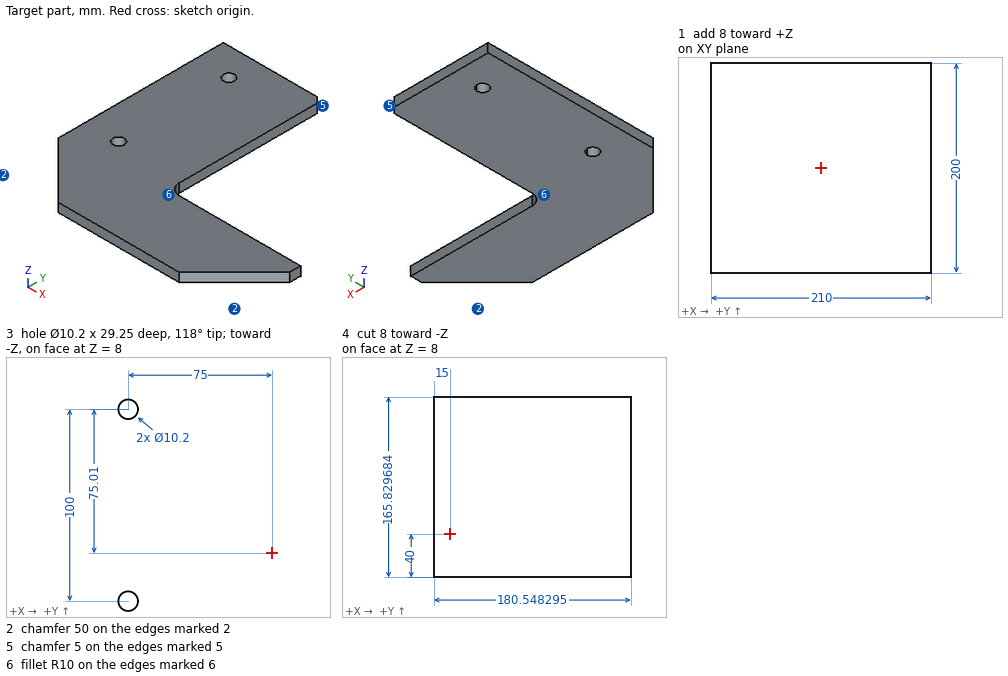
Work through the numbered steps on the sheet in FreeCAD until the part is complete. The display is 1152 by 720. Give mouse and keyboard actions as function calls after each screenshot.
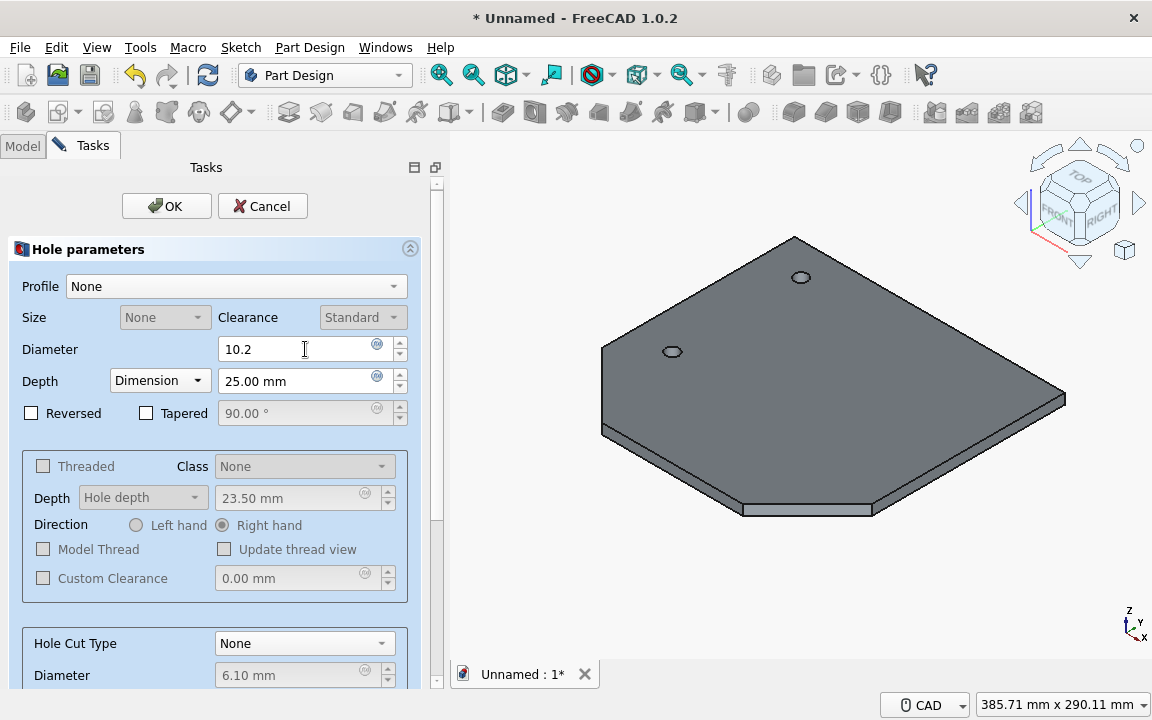
triple_click(305, 381)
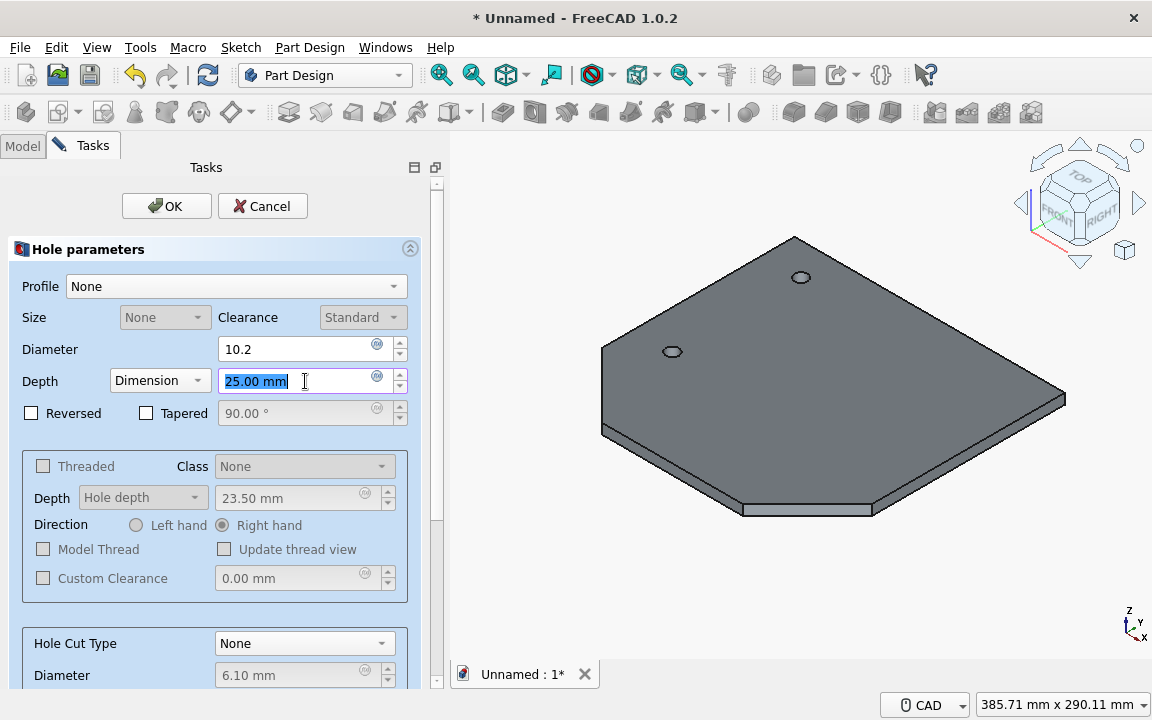
text(29.25)
key(Tab)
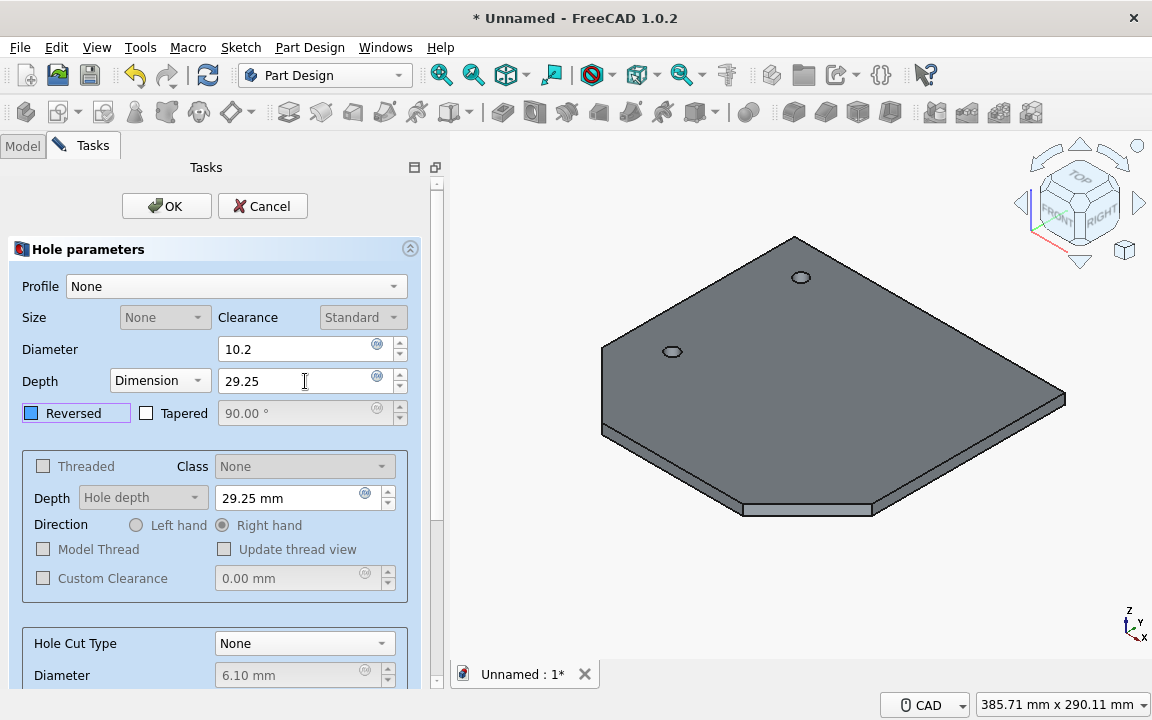
click(167, 206)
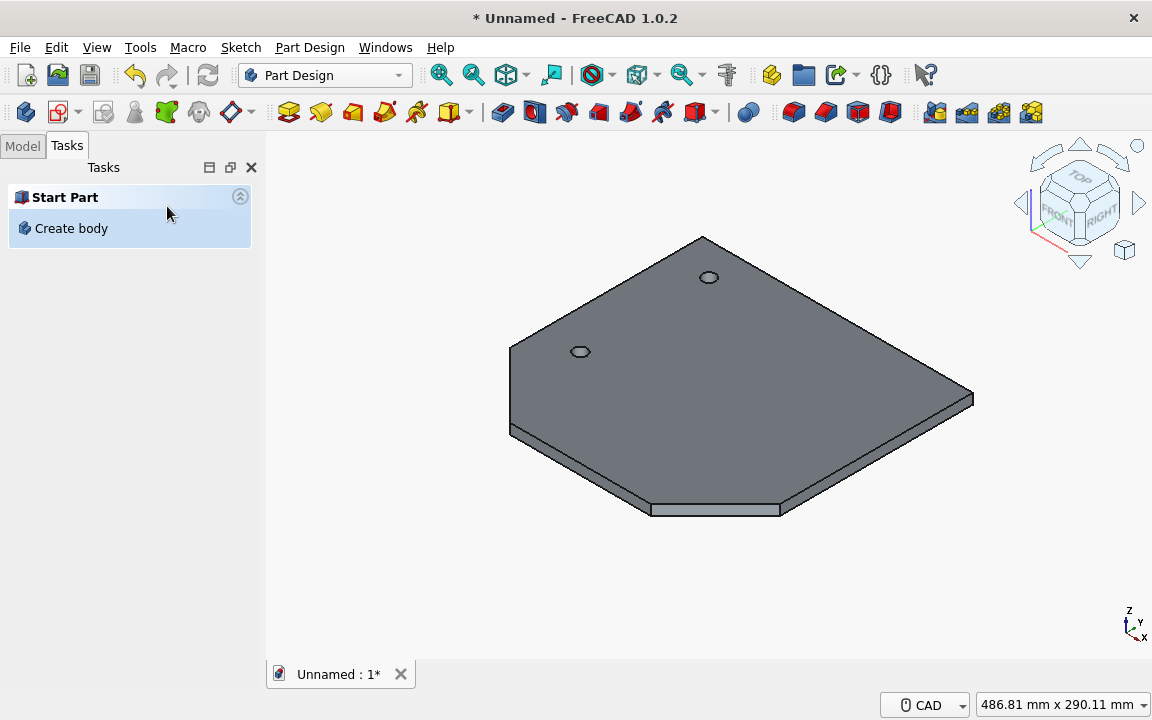
click(748, 410)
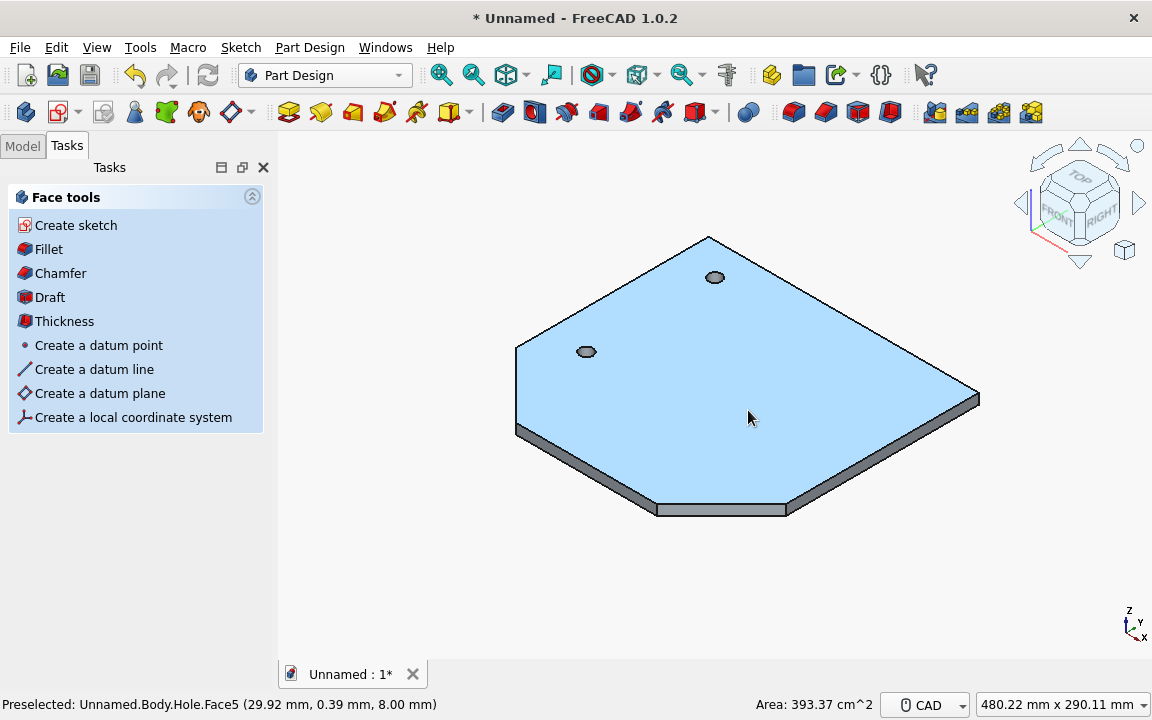
click(58, 112)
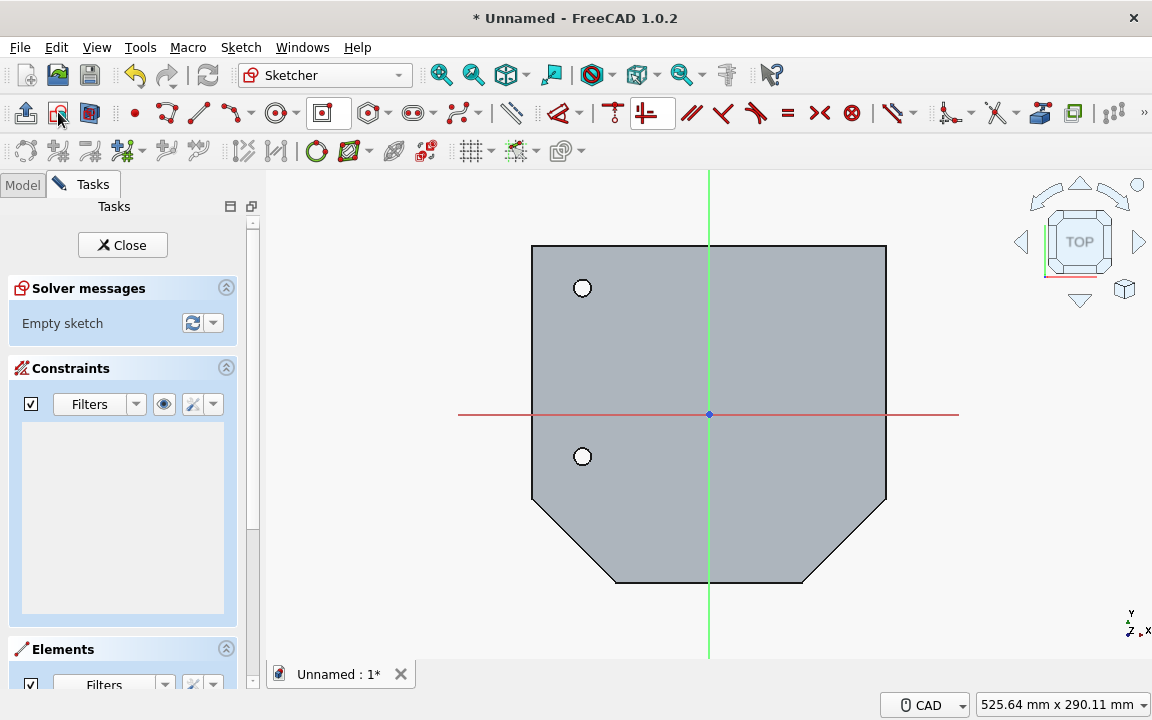
scroll(294, 631, down, 1)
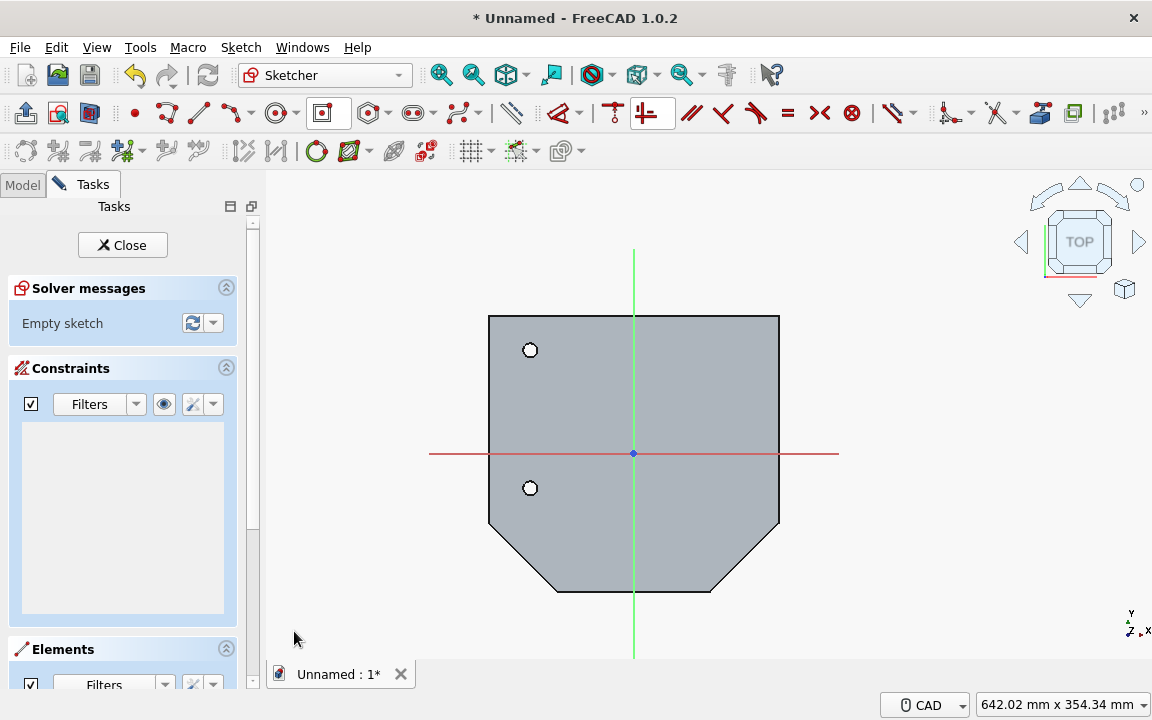
key(g)
key(r)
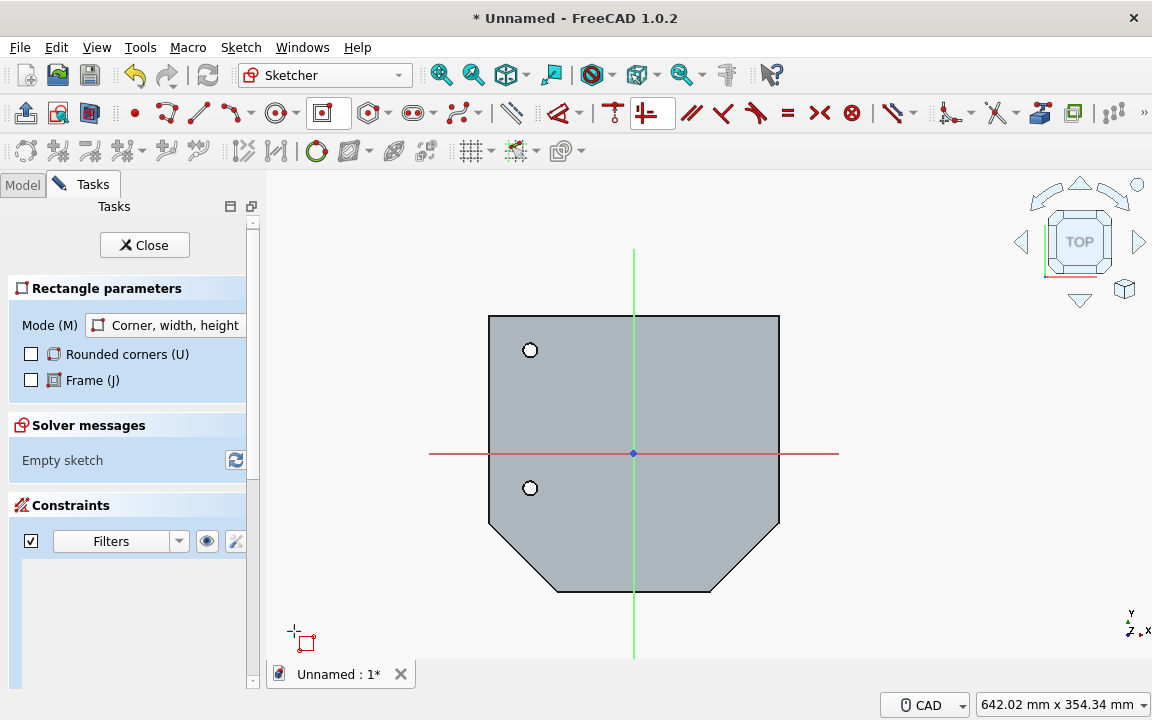
click(613, 280)
click(862, 509)
key(Escape)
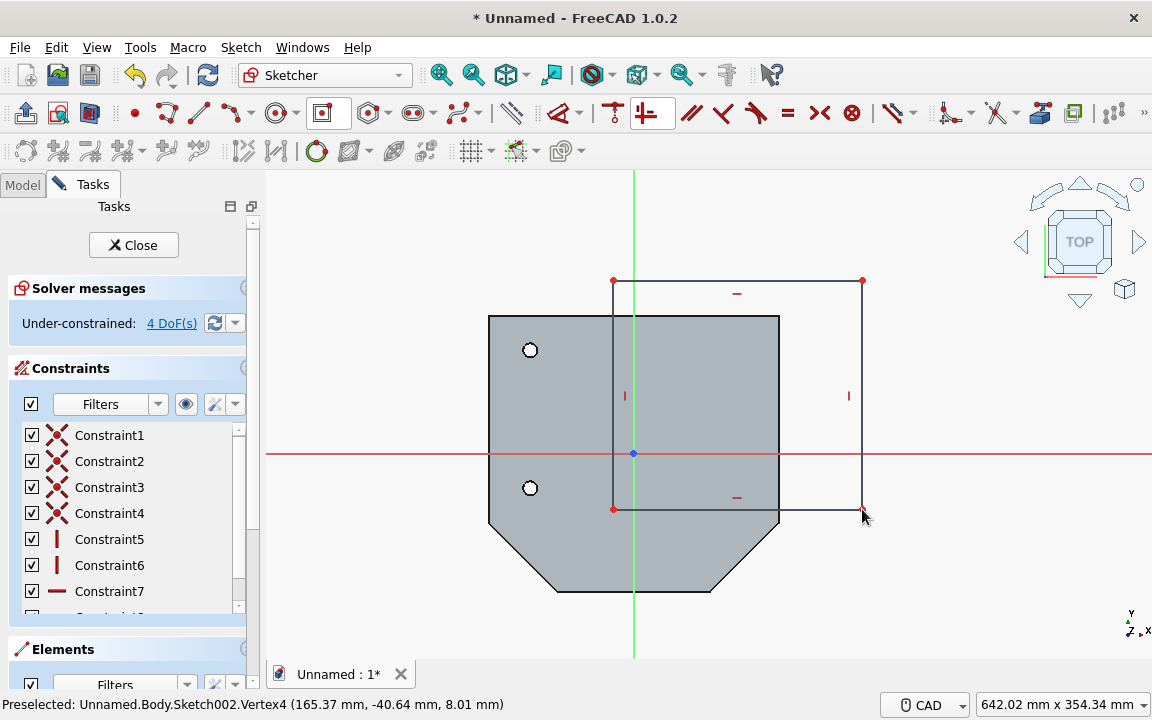
scroll(613, 281, up, 4)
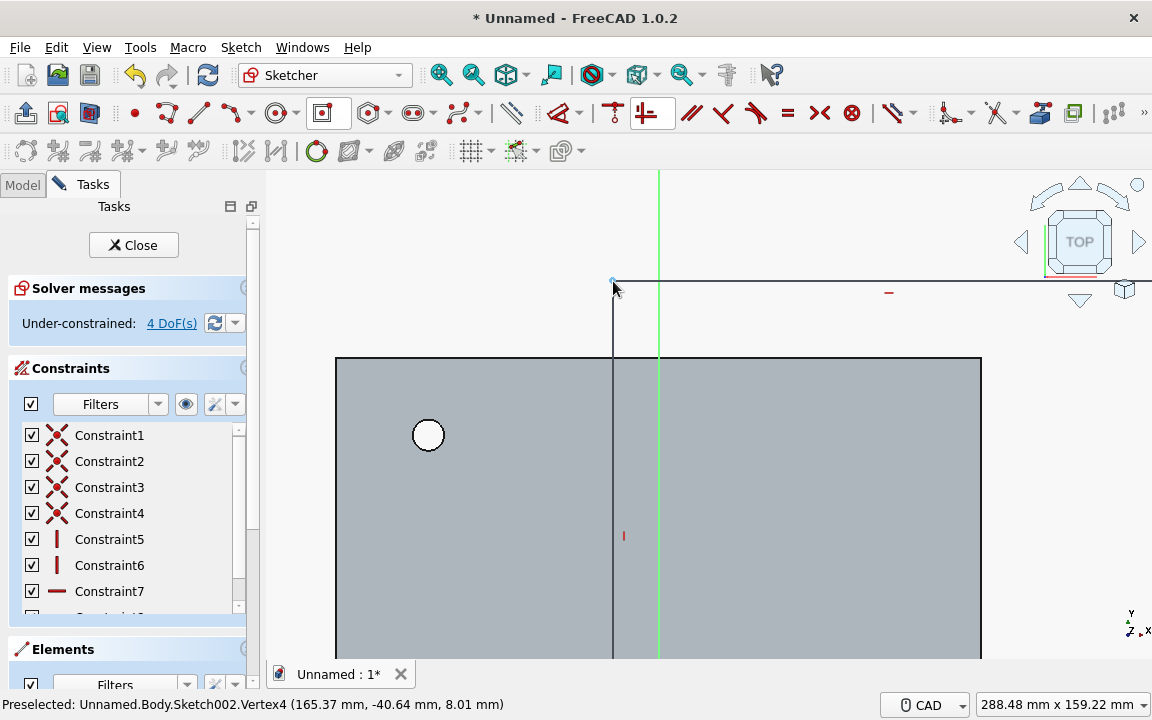
click(613, 281)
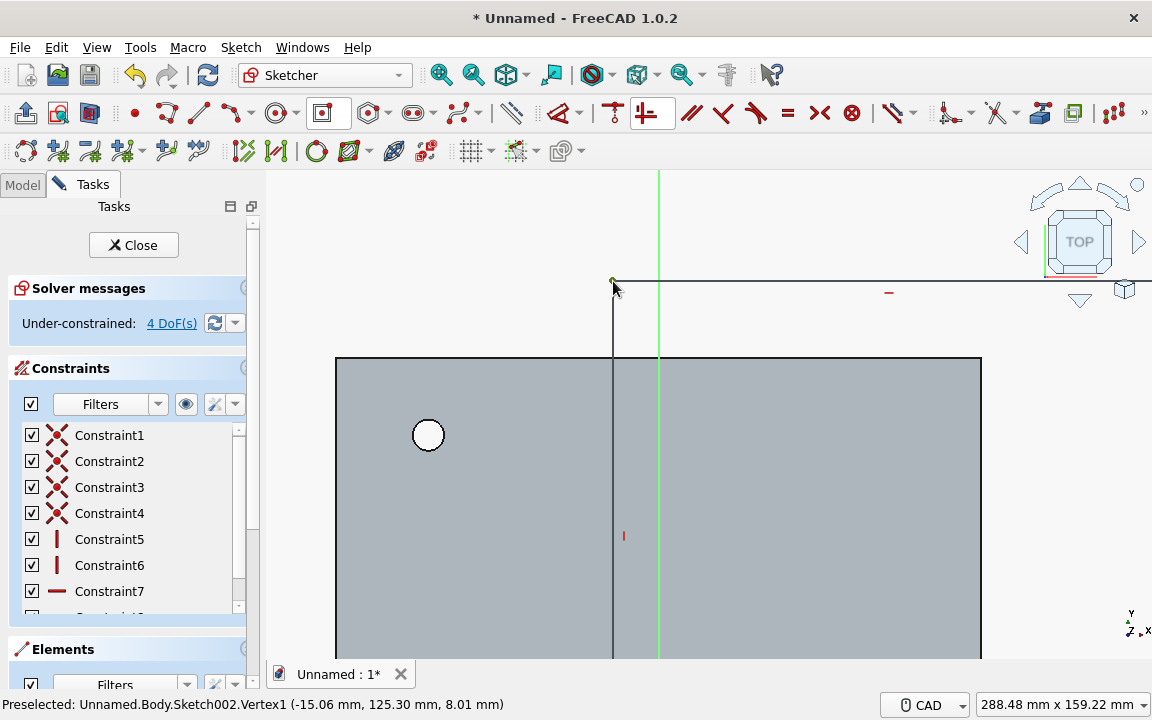
key(l)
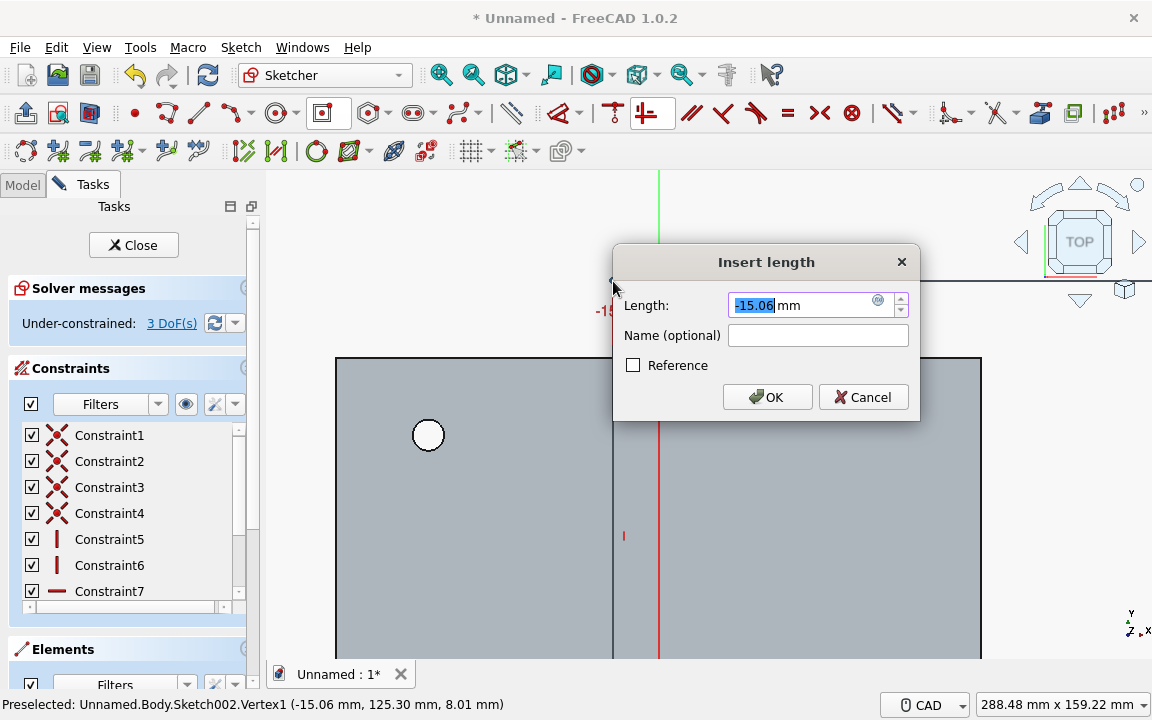
text(-15)
key(Return)